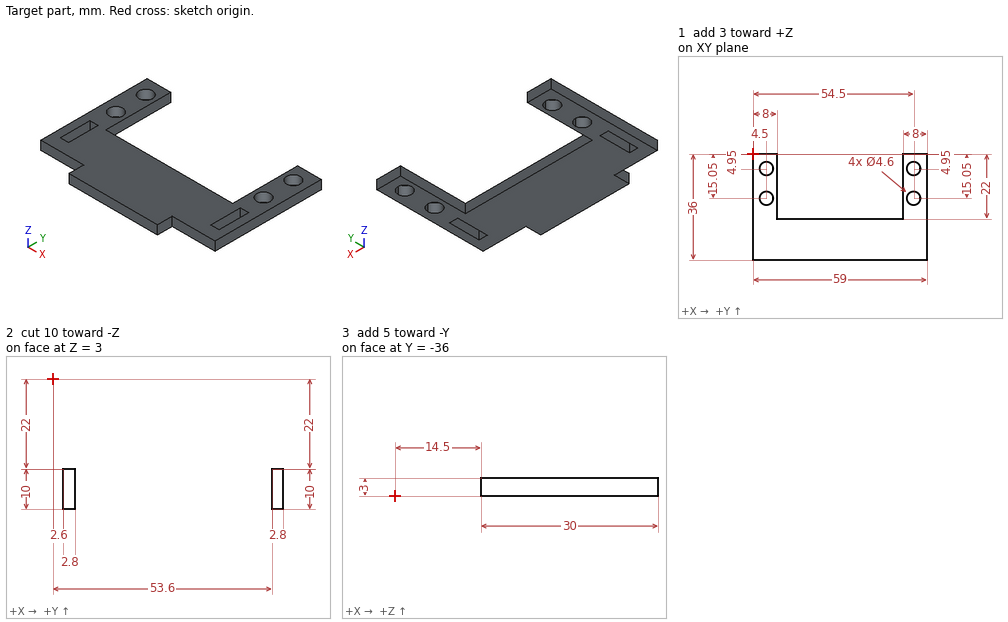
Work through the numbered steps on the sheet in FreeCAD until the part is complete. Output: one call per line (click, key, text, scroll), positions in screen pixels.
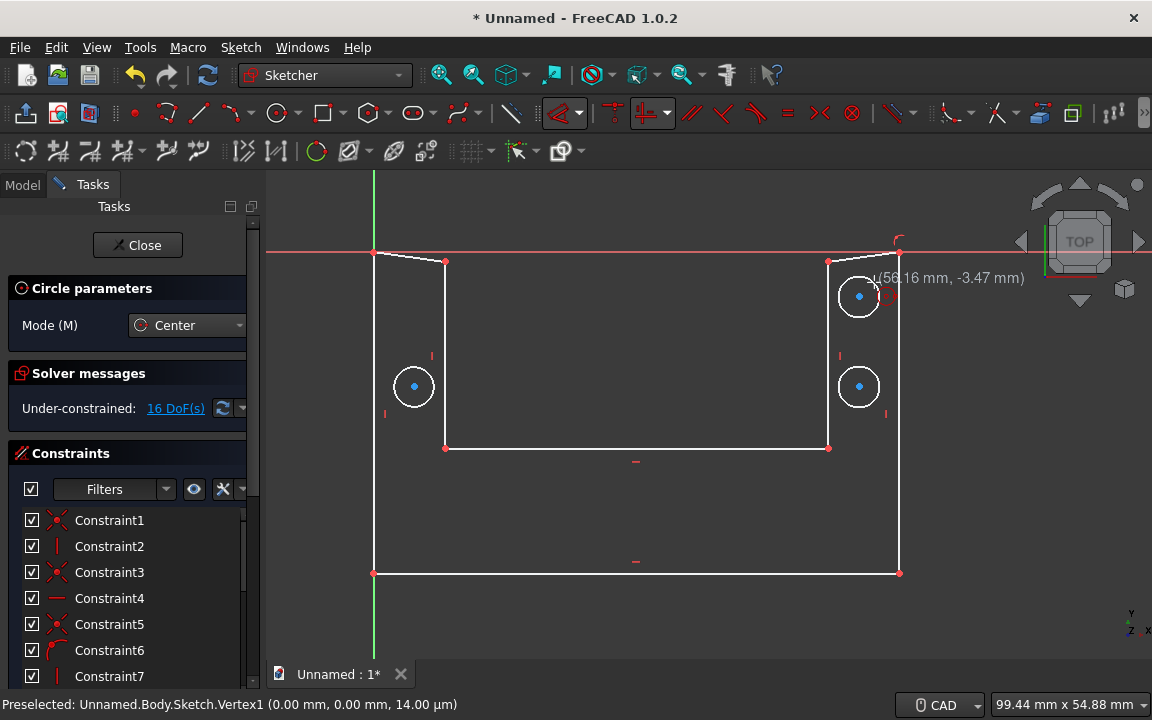
click(414, 296)
click(428, 282)
key(Escape)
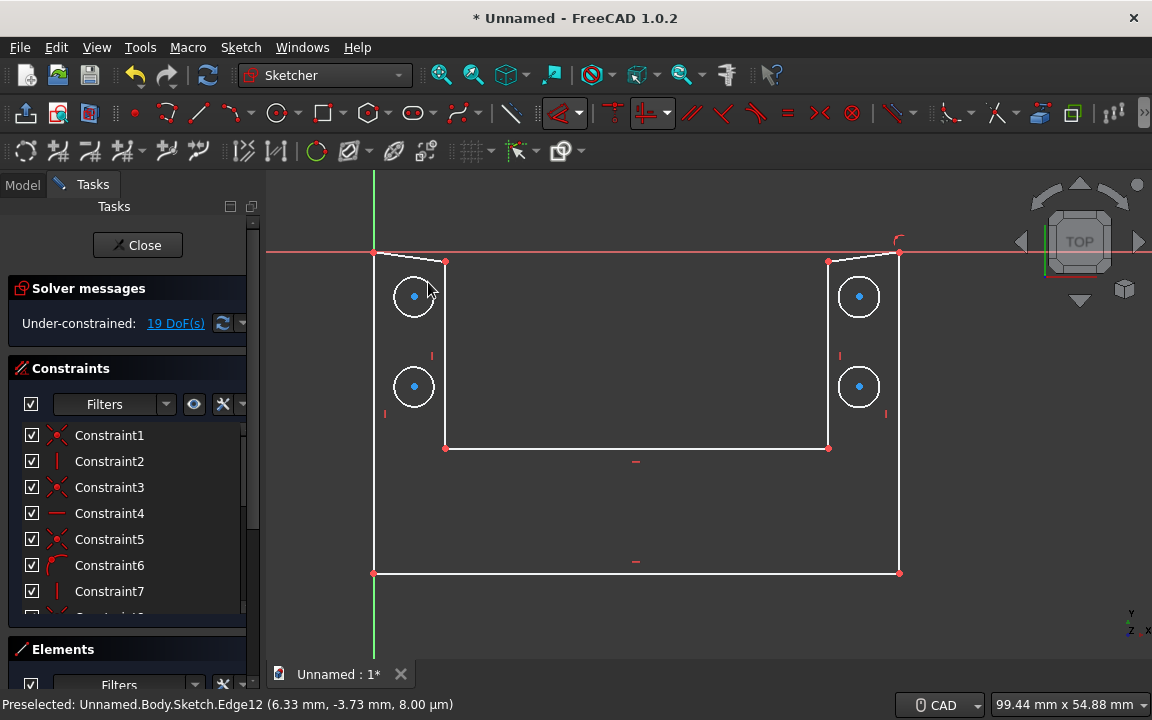
click(878, 255)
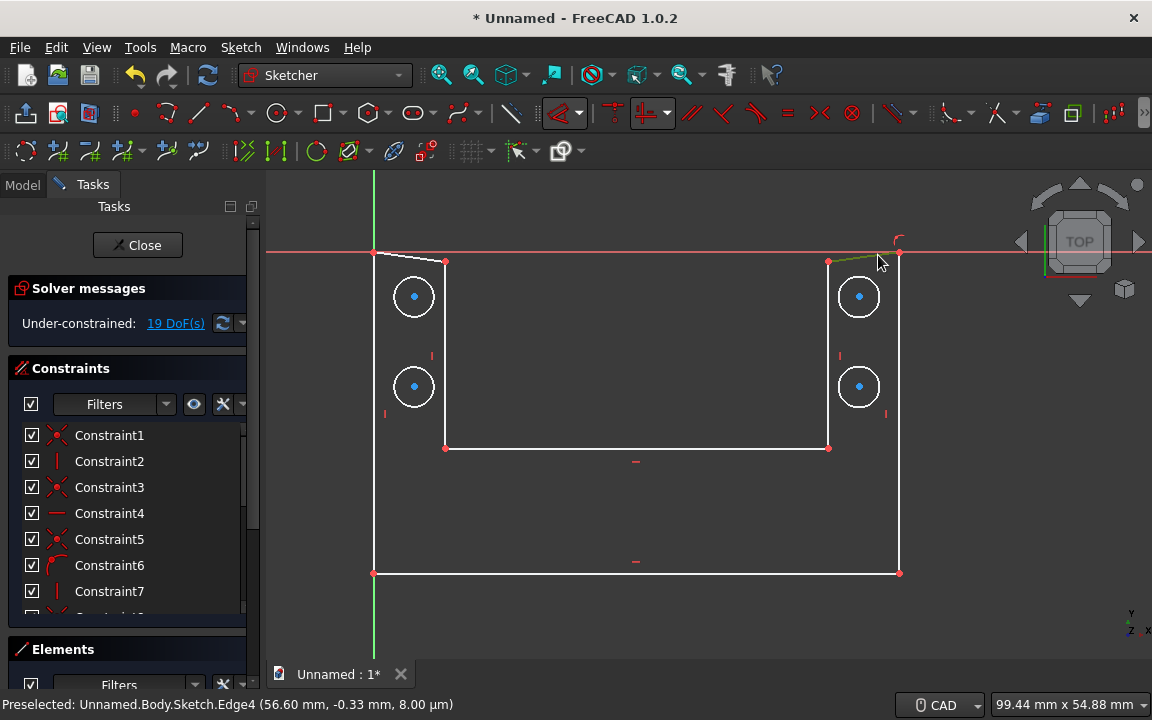
key(h)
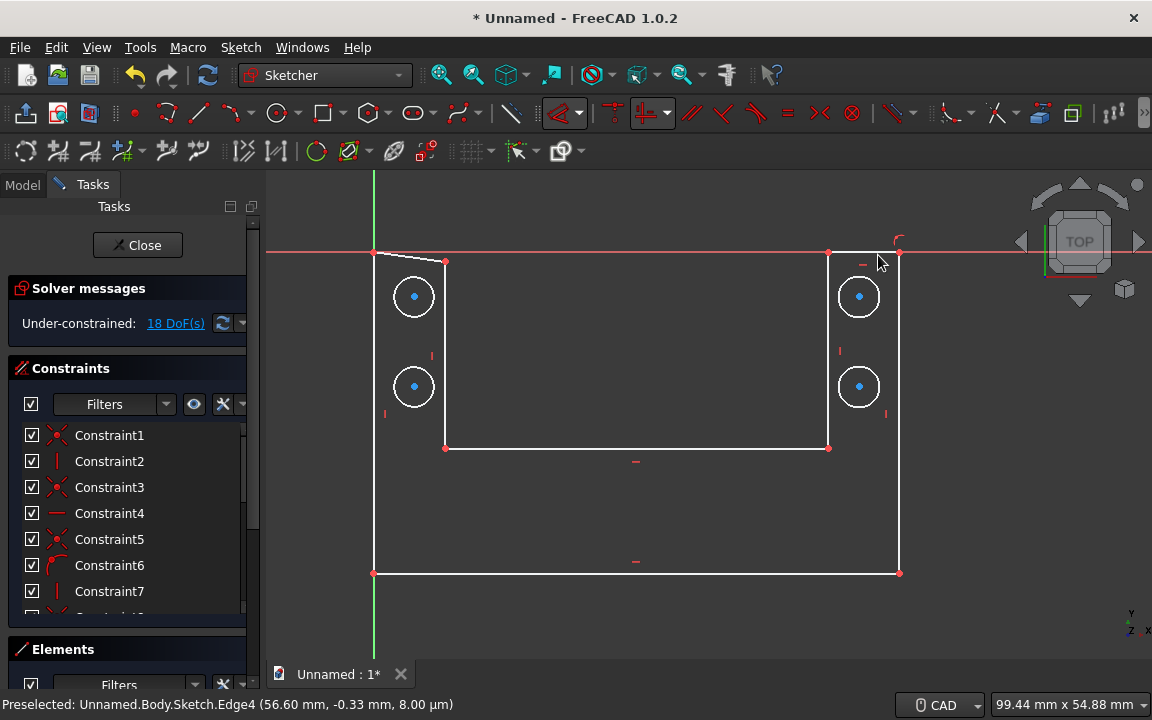
click(395, 255)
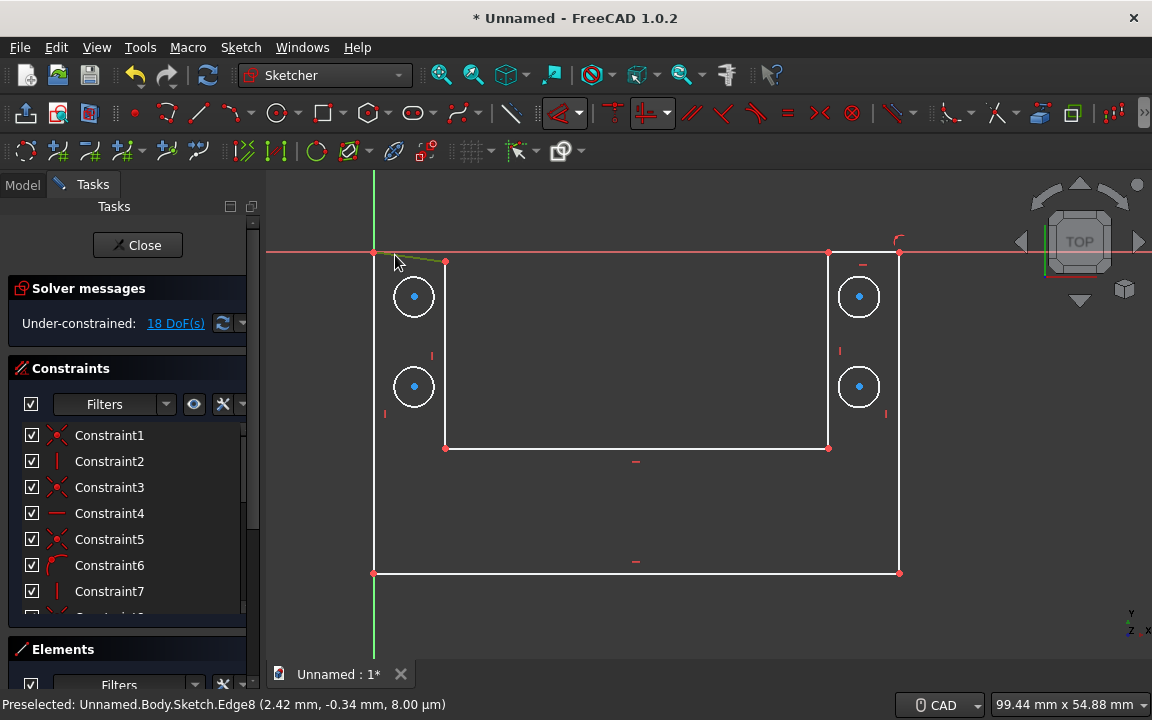
key(h)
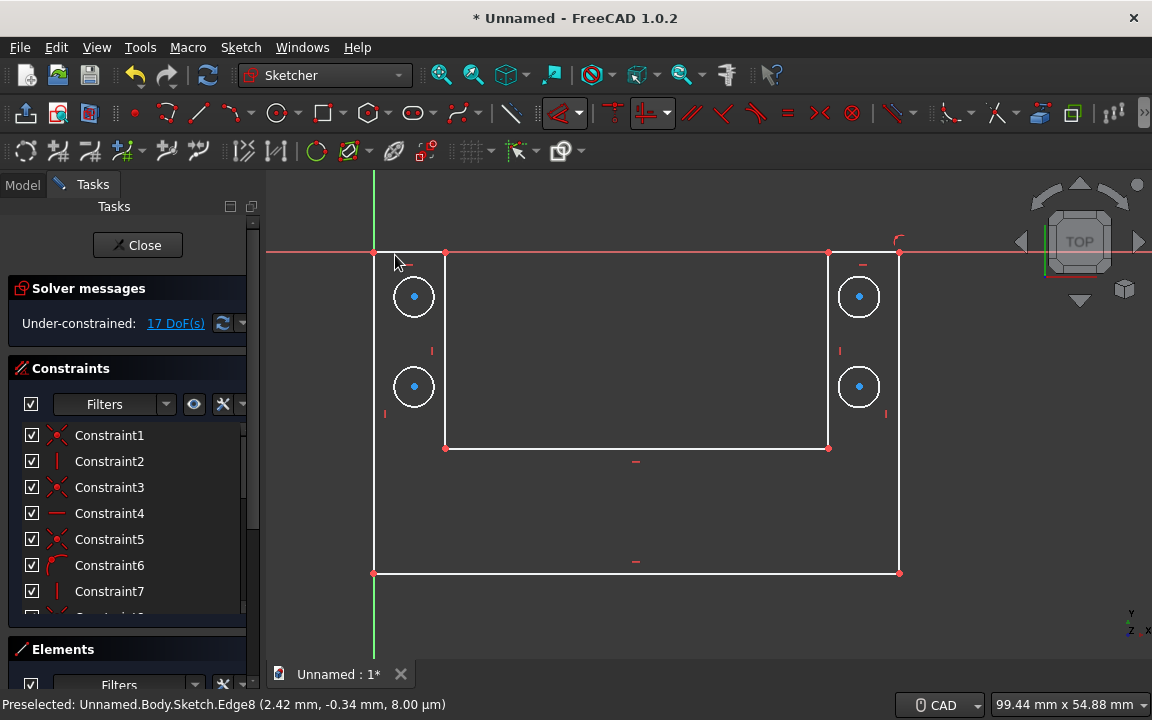
click(873, 372)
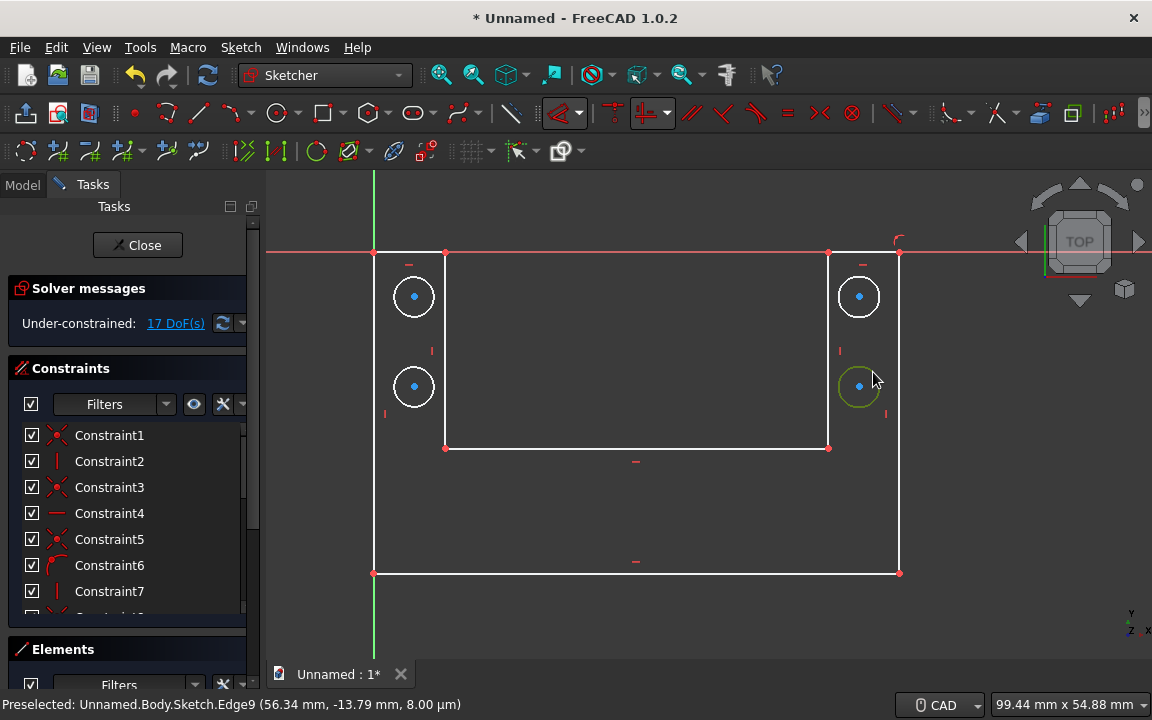
click(428, 373)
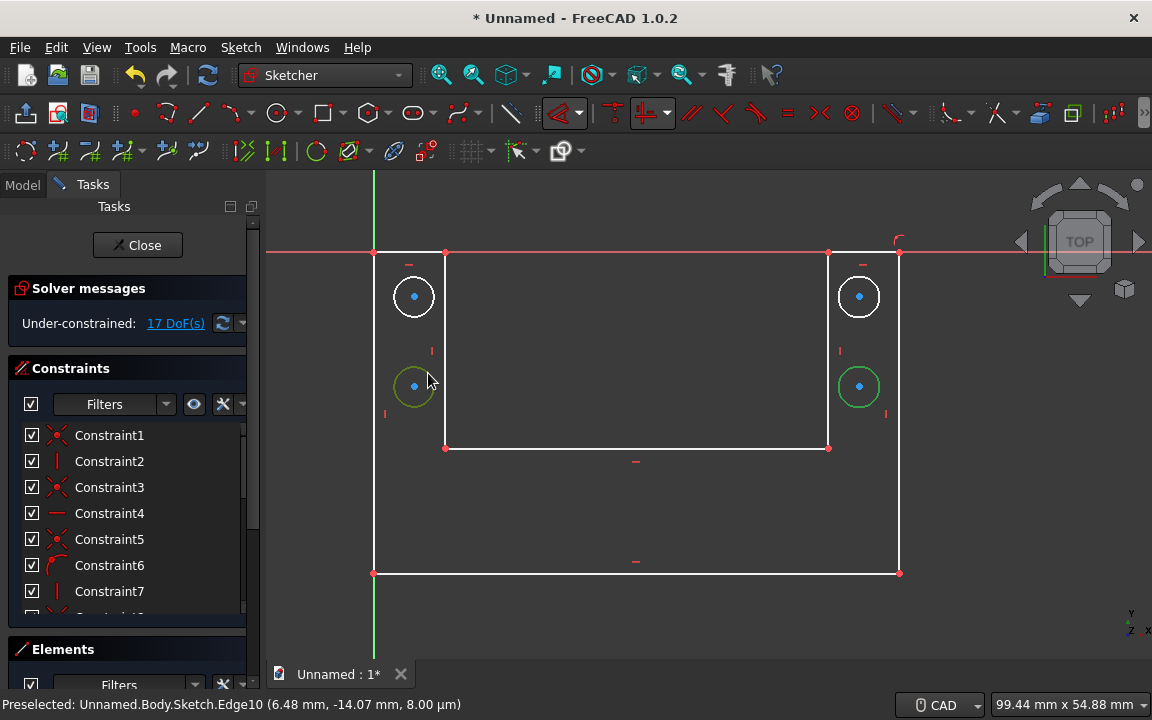
click(873, 282)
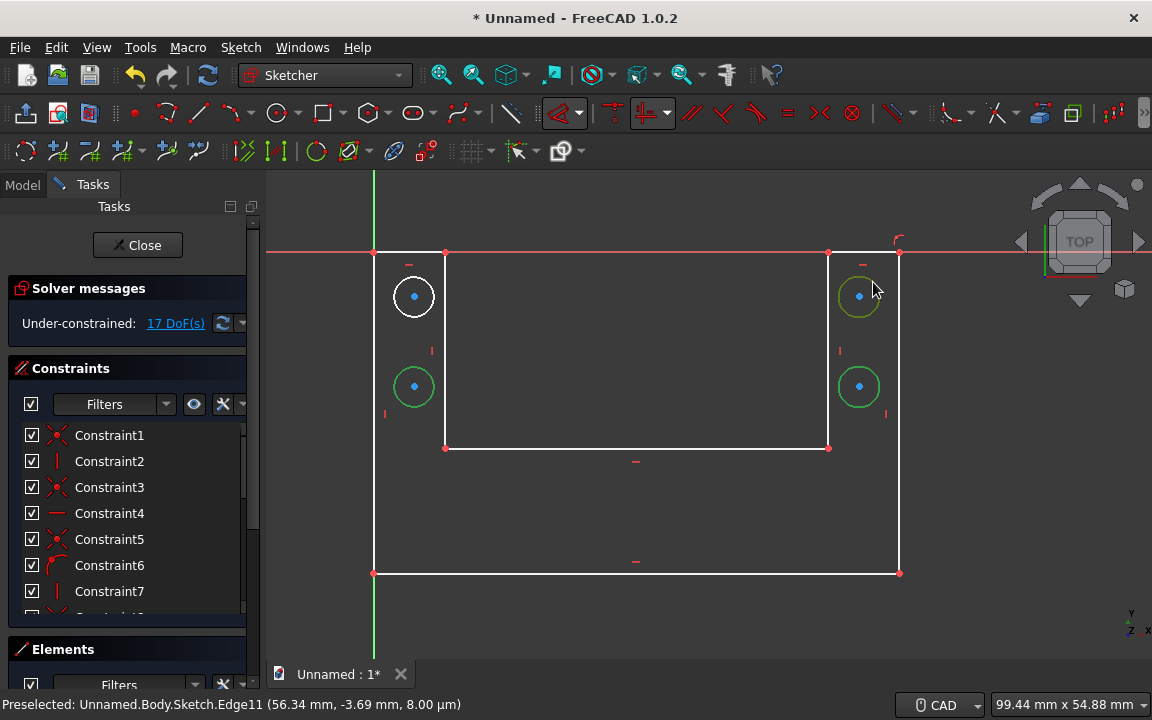
click(428, 283)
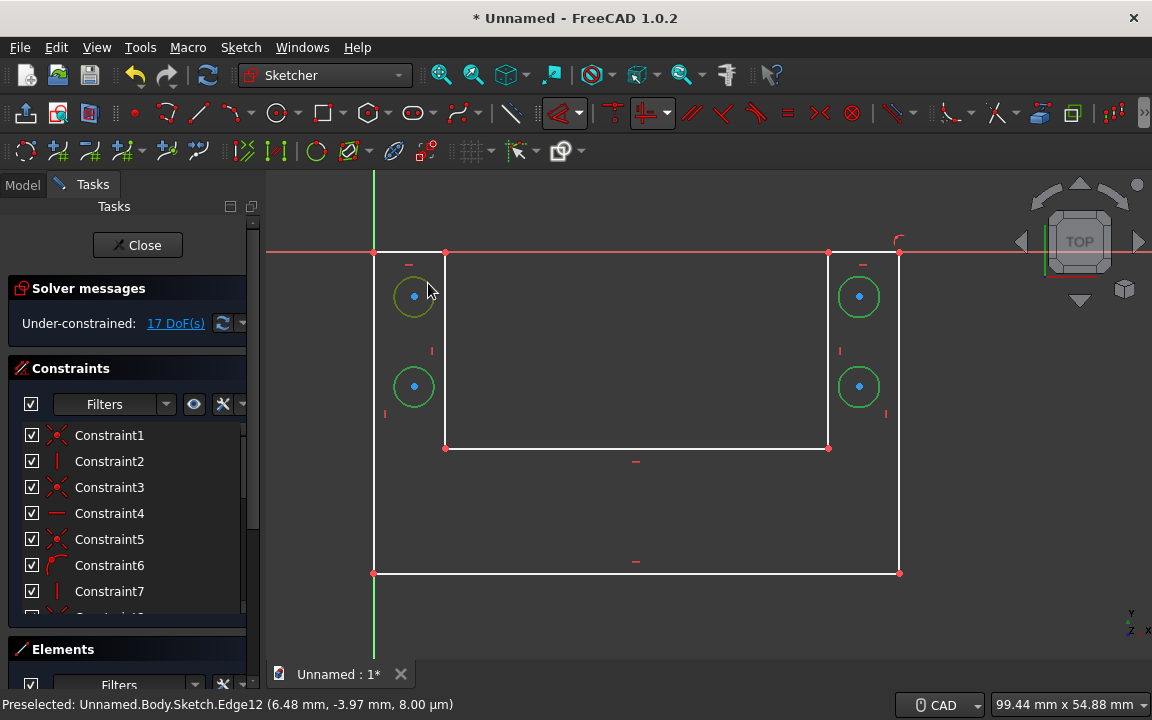
key(e)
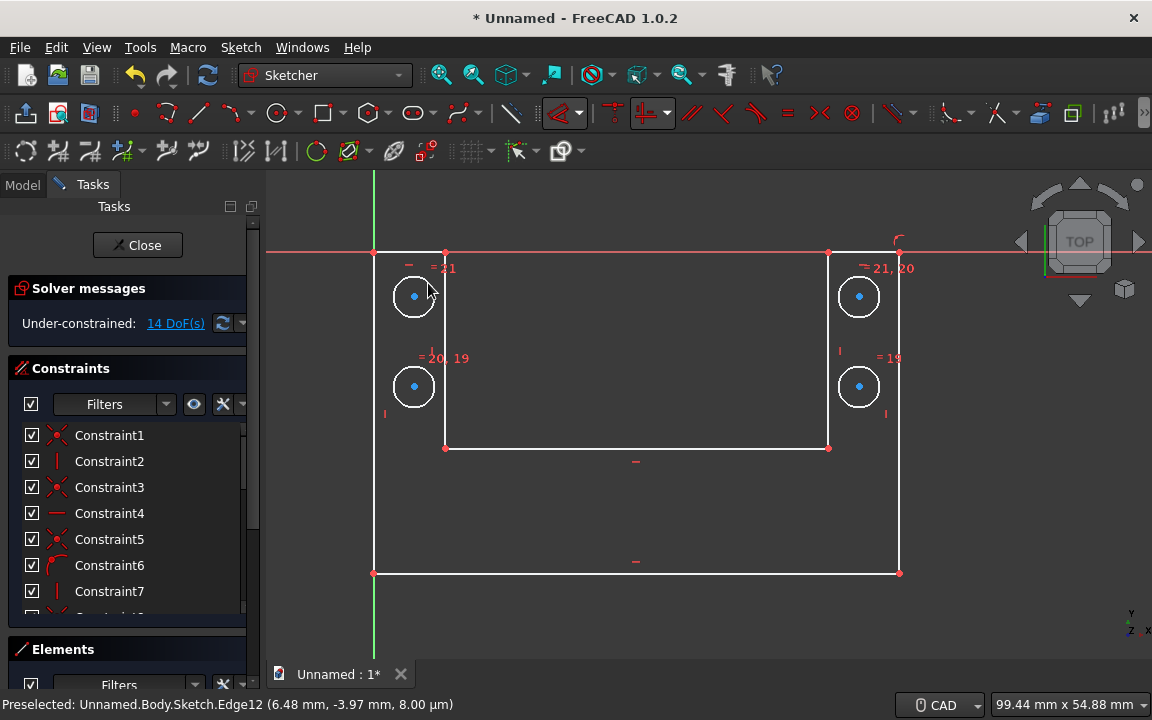
click(859, 387)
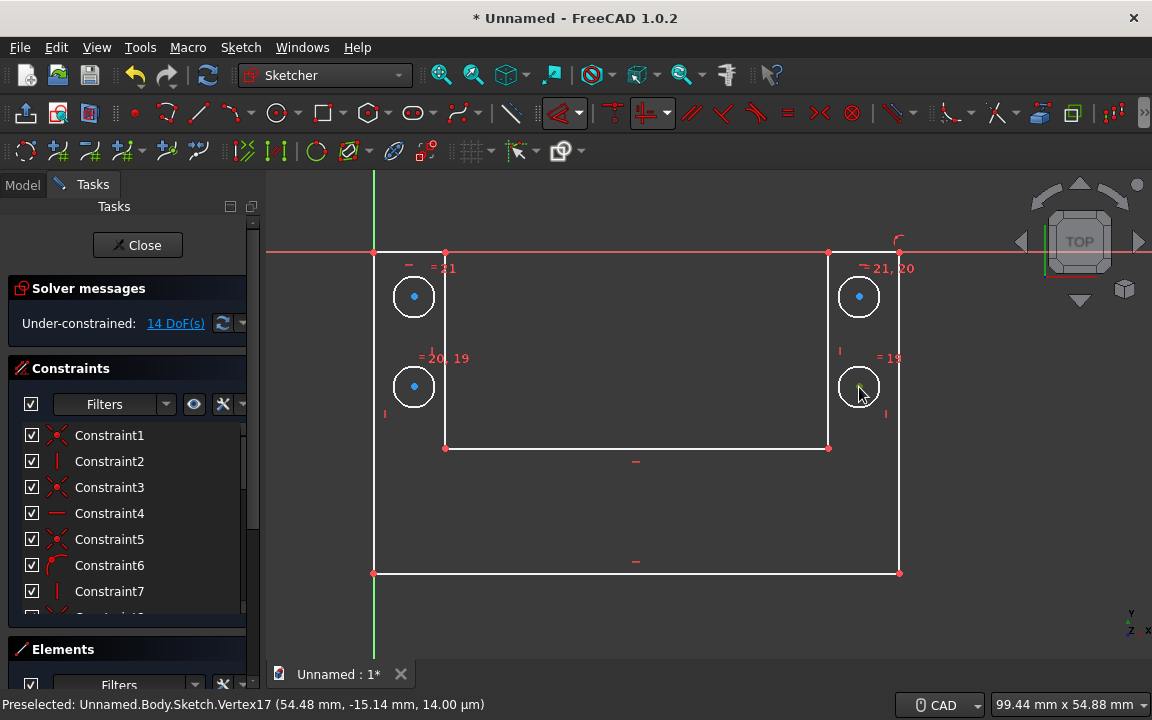
click(859, 297)